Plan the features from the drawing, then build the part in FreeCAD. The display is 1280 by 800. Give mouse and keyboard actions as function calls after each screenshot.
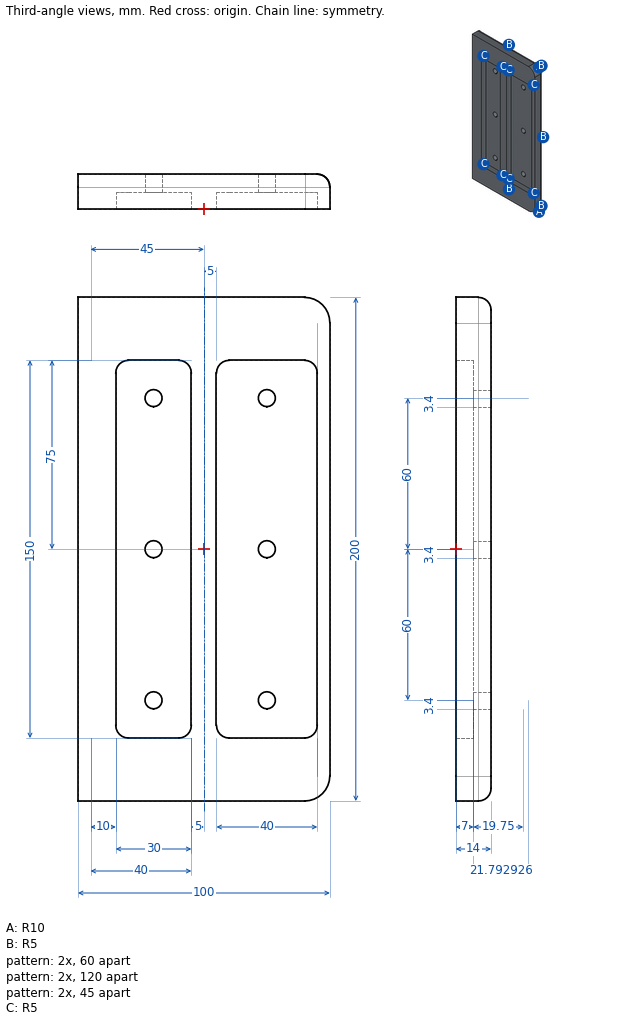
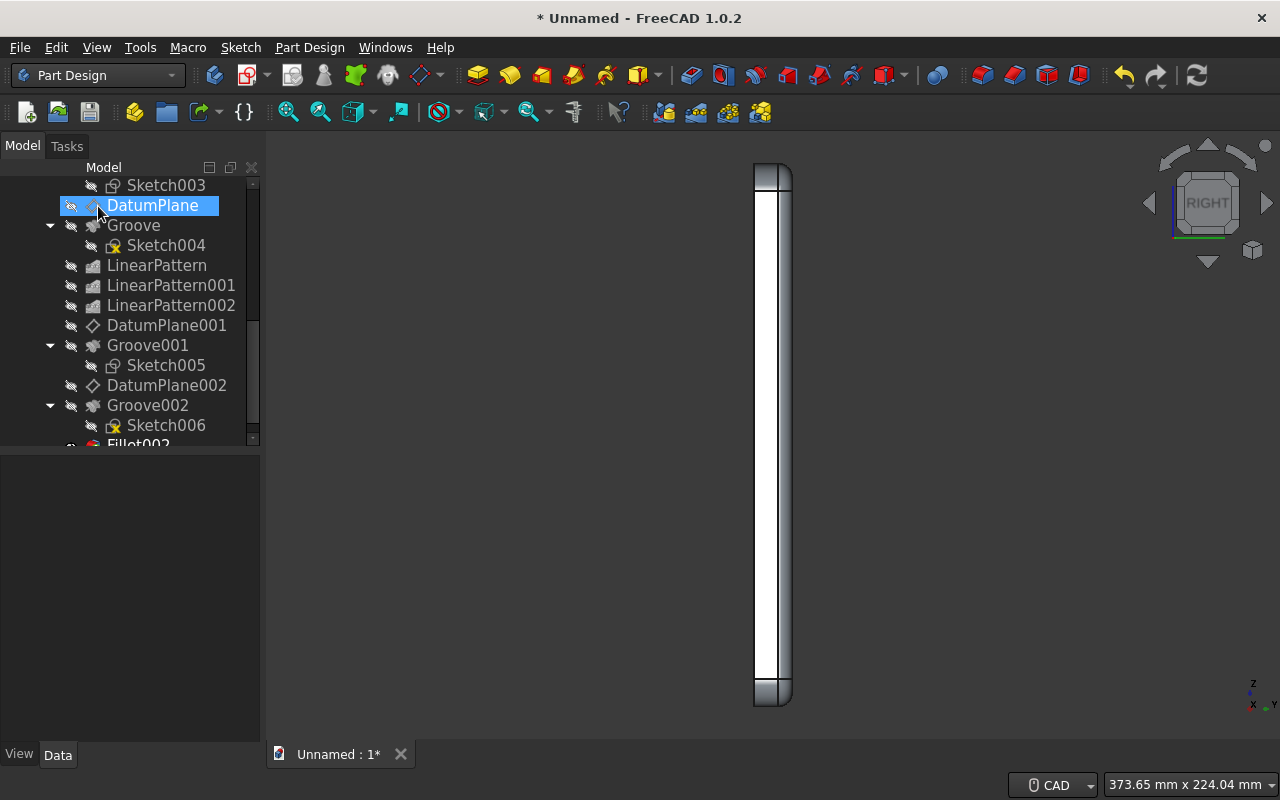
key(0)